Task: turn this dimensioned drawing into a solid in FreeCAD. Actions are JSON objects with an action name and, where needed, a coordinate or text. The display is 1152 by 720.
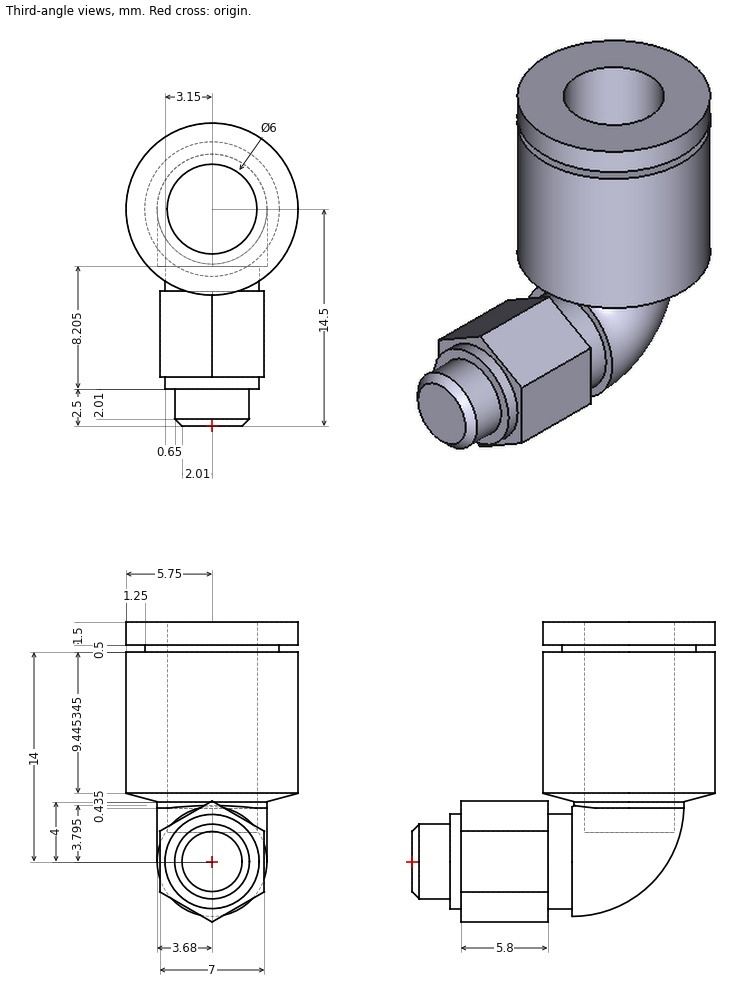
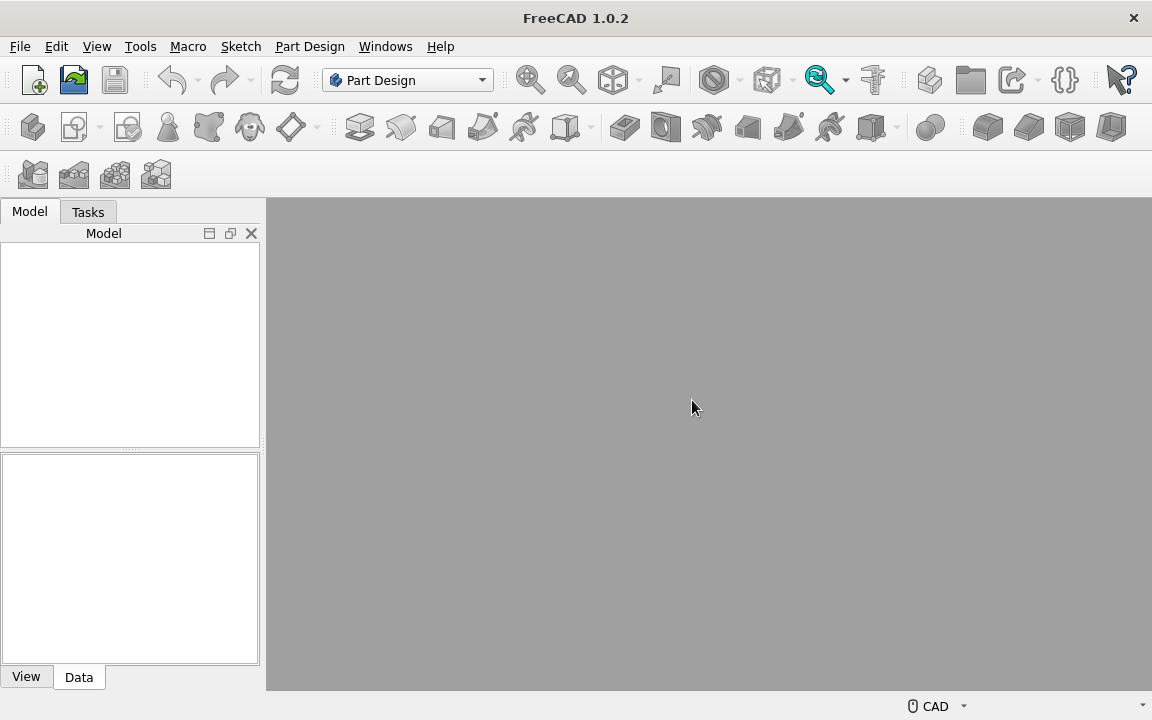
{"action": "left_click", "coordinate": [33, 80]}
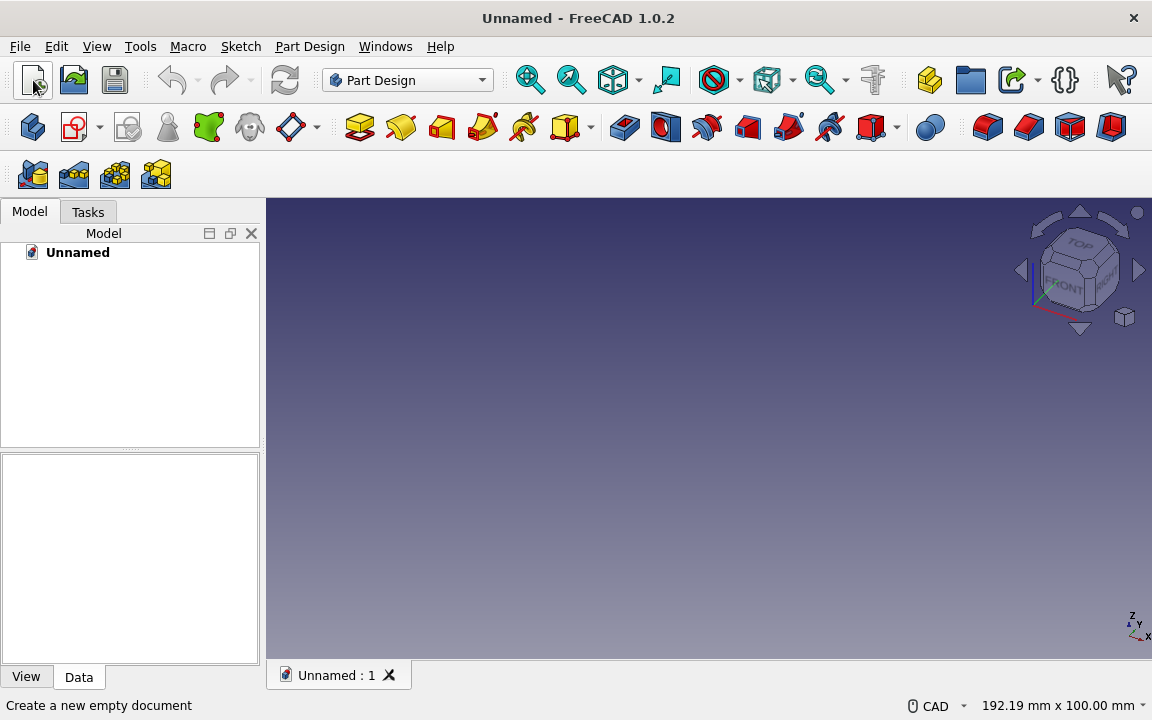
{"action": "left_click", "coordinate": [74, 128]}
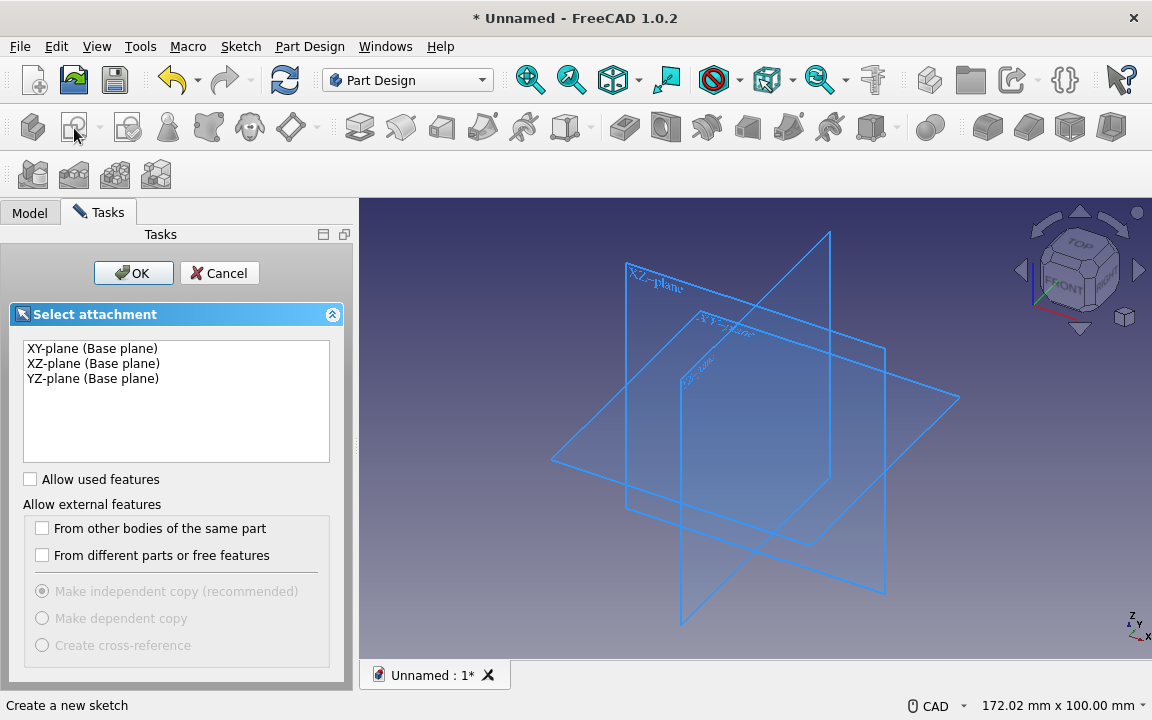
{"action": "left_click", "coordinate": [84, 348]}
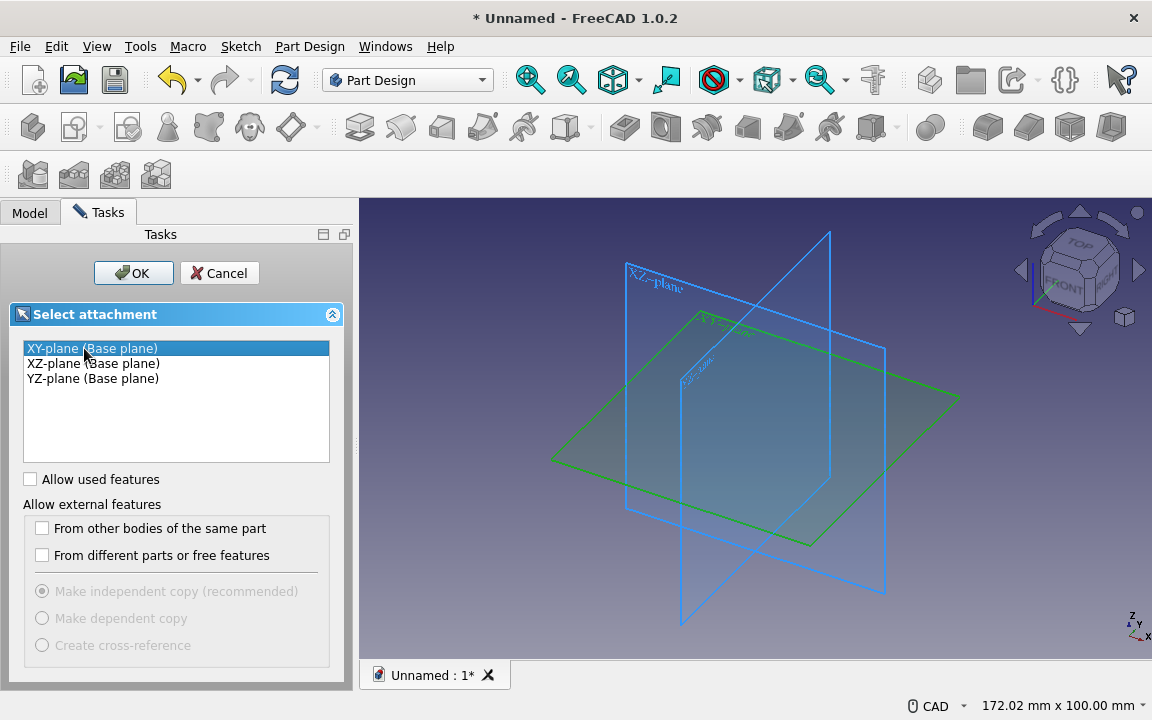
{"action": "left_click", "coordinate": [134, 273]}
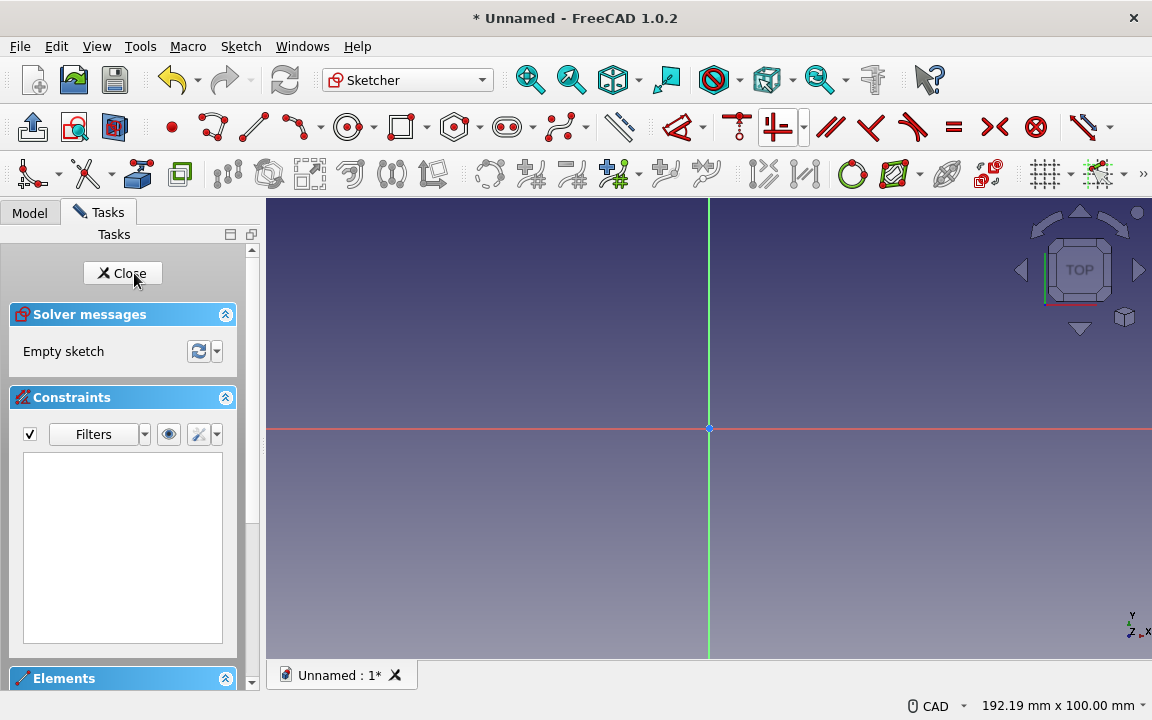
{"action": "scroll", "coordinate": [714, 399], "scroll_direction": "up", "scroll_amount": 9}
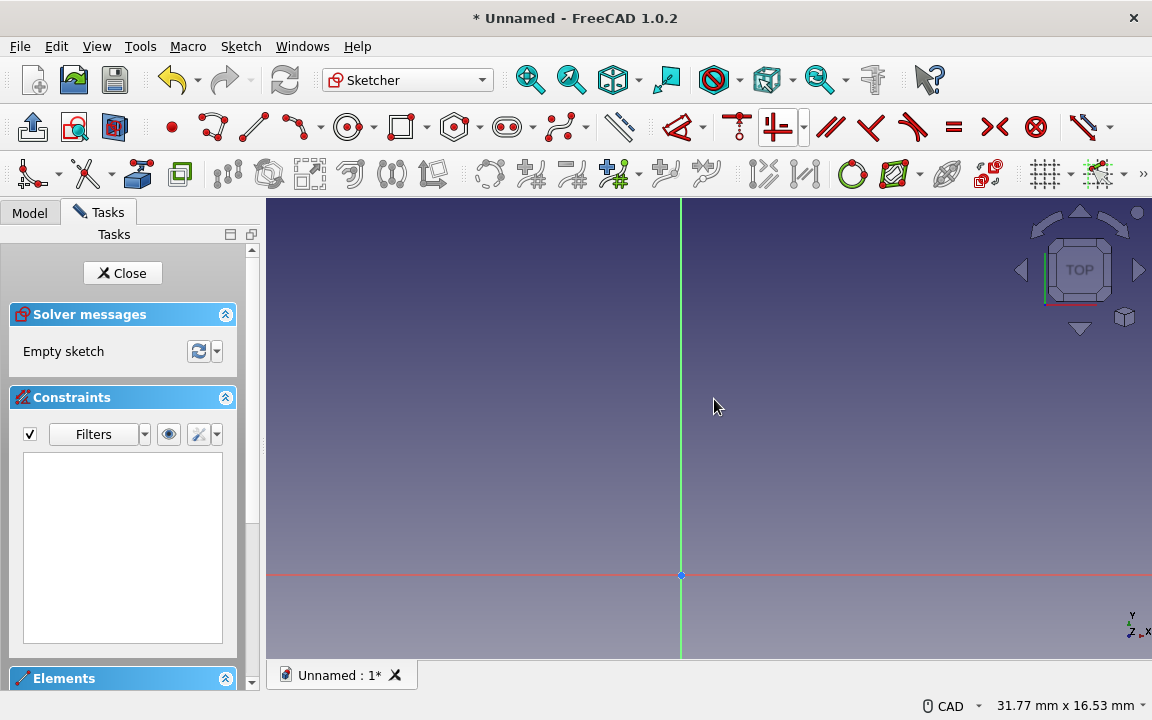
{"action": "left_click", "coordinate": [213, 128]}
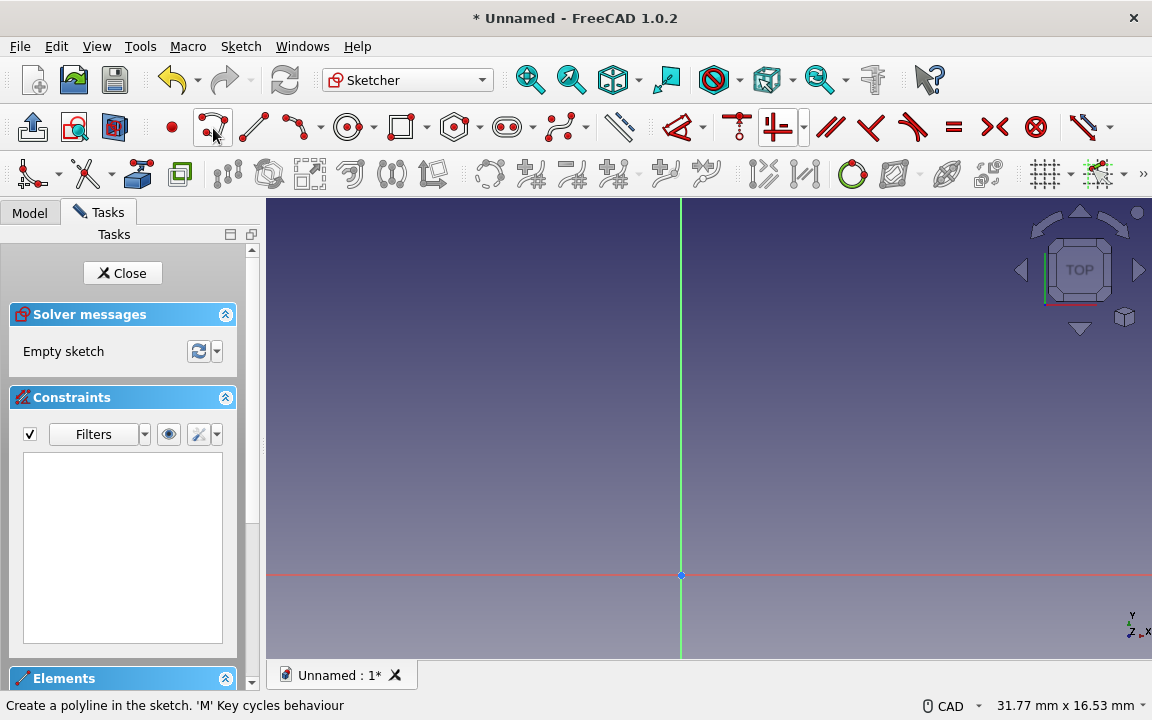
{"action": "left_click", "coordinate": [681, 575]}
{"action": "left_click", "coordinate": [672, 277]}
{"action": "left_click", "coordinate": [593, 277]}
{"action": "left_click", "coordinate": [593, 506]}
{"action": "left_click", "coordinate": [611, 506]}
{"action": "left_click", "coordinate": [611, 562]}
{"action": "left_click", "coordinate": [625, 566]}
{"action": "left_click", "coordinate": [681, 575]}
{"action": "key", "text": "Escape"}
{"action": "key", "text": "Escape"}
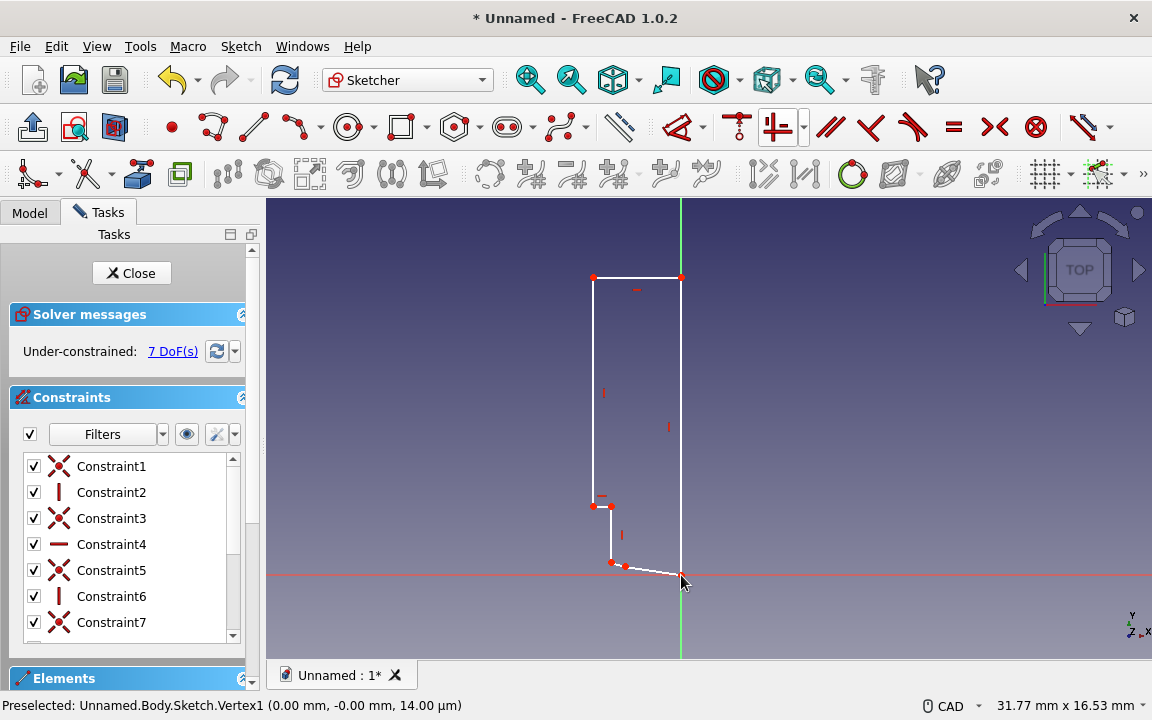
{"action": "left_click", "coordinate": [664, 573]}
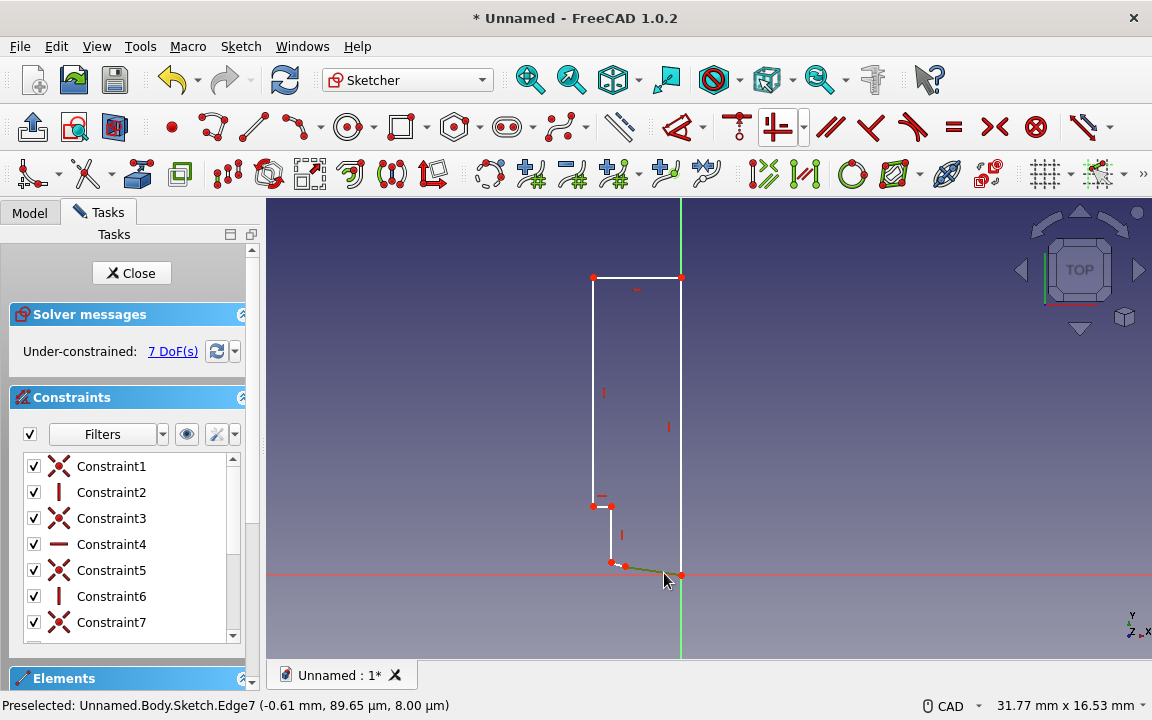
{"action": "left_click", "coordinate": [804, 128]}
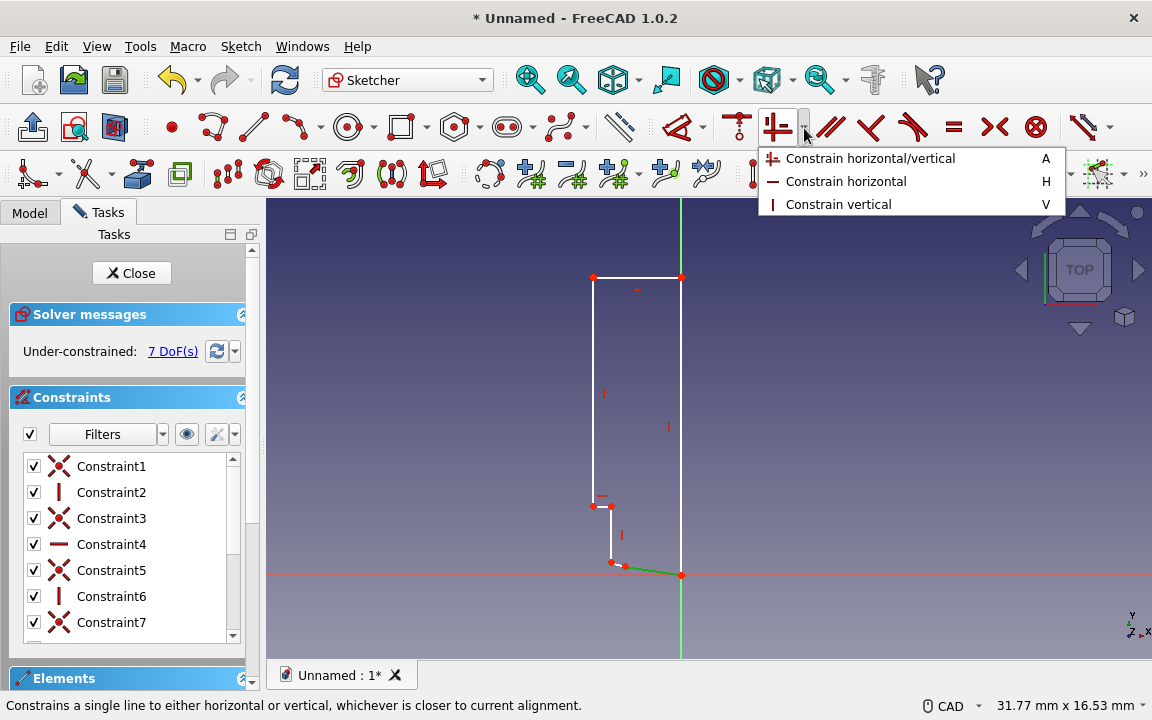
{"action": "left_click", "coordinate": [912, 182]}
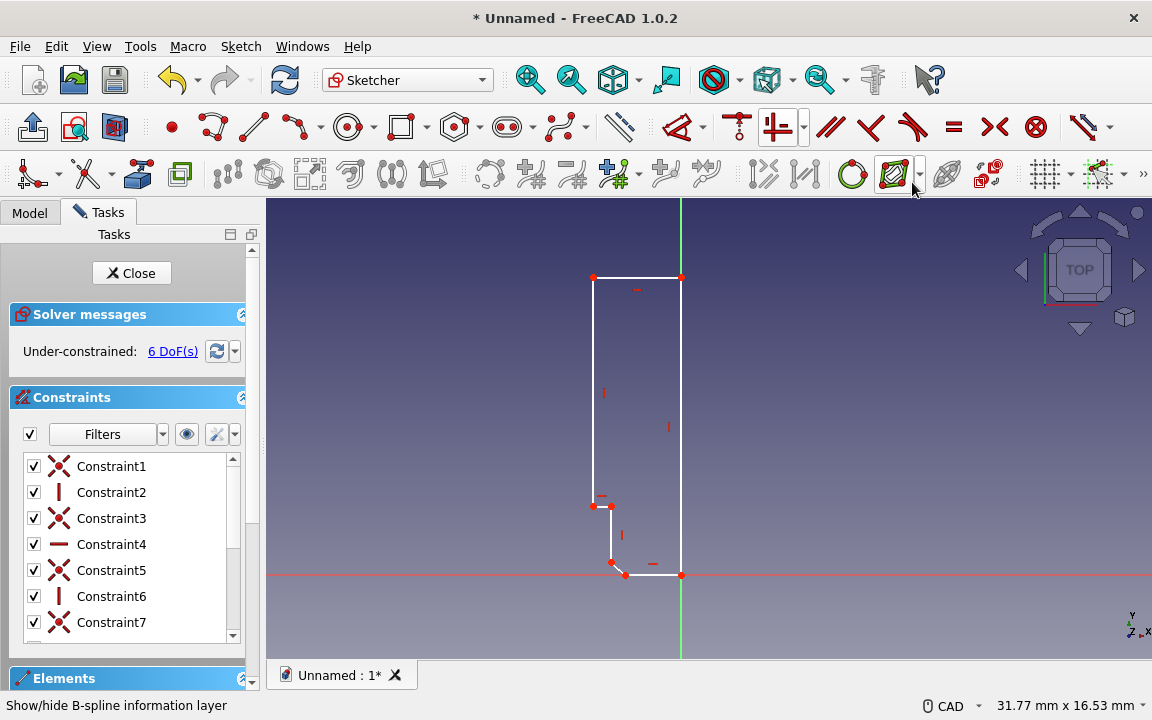
{"action": "left_click", "coordinate": [655, 278]}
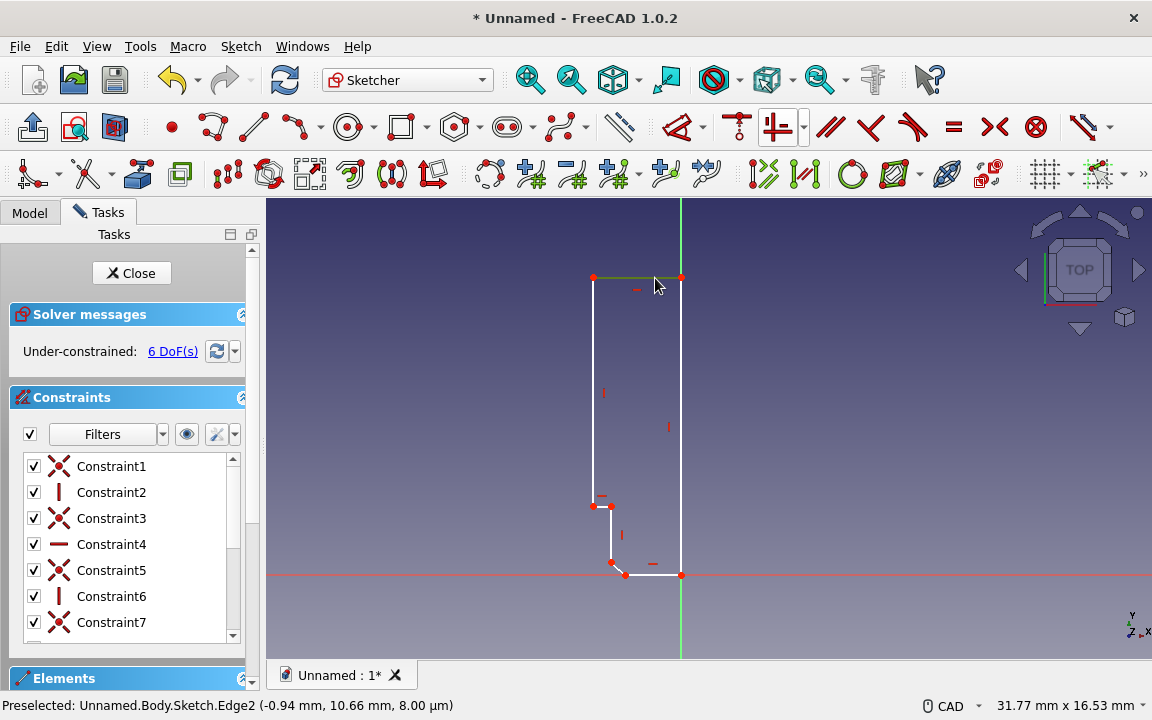
{"action": "left_click", "coordinate": [702, 128]}